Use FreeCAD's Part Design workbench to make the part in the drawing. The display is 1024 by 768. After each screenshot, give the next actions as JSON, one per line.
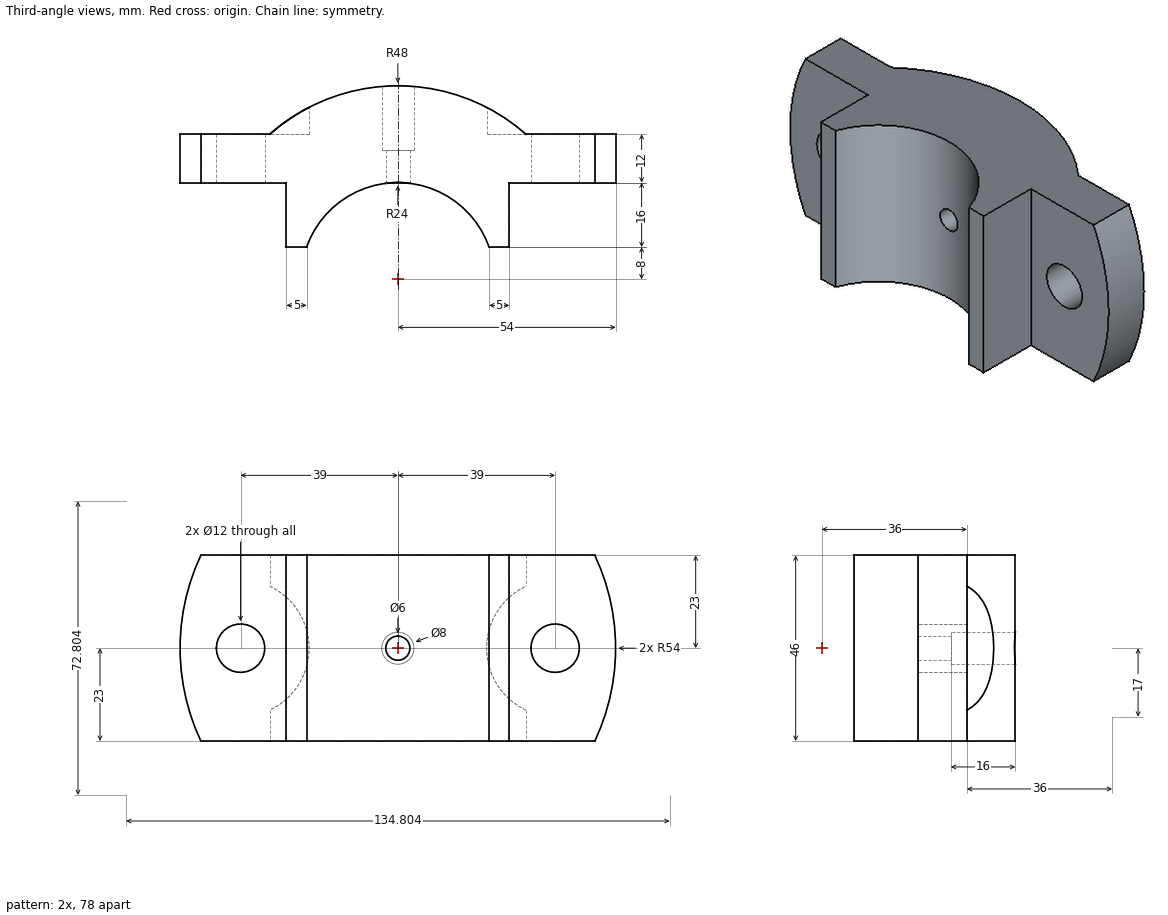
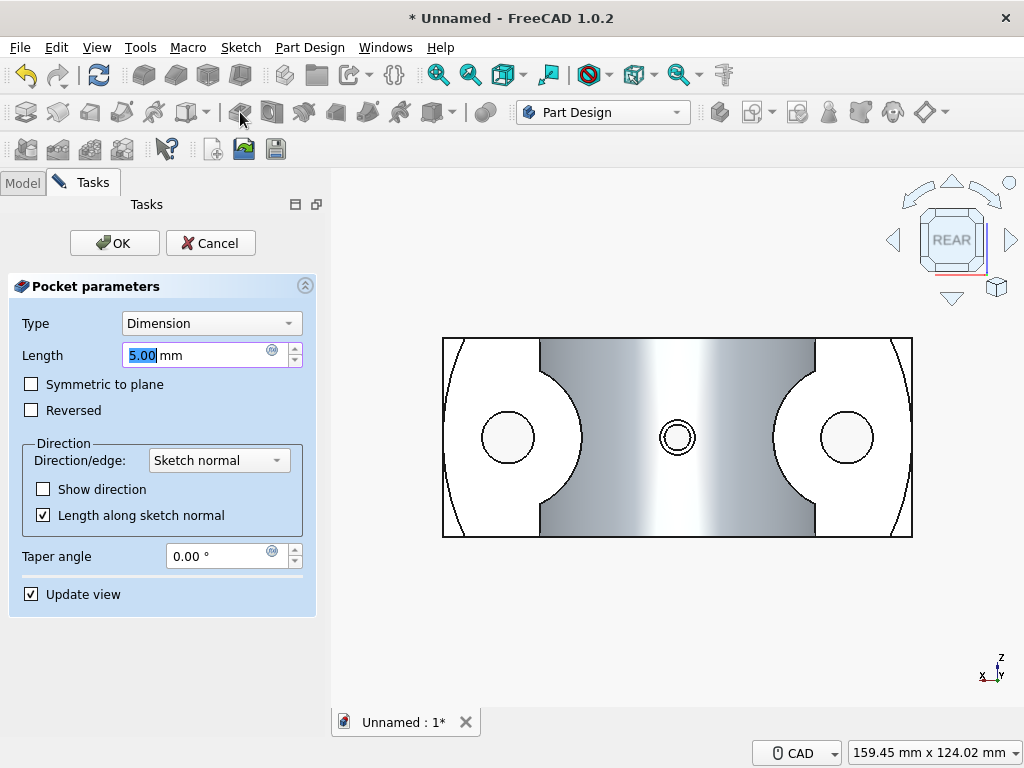
{"action": "left_click", "coordinate": [212, 324]}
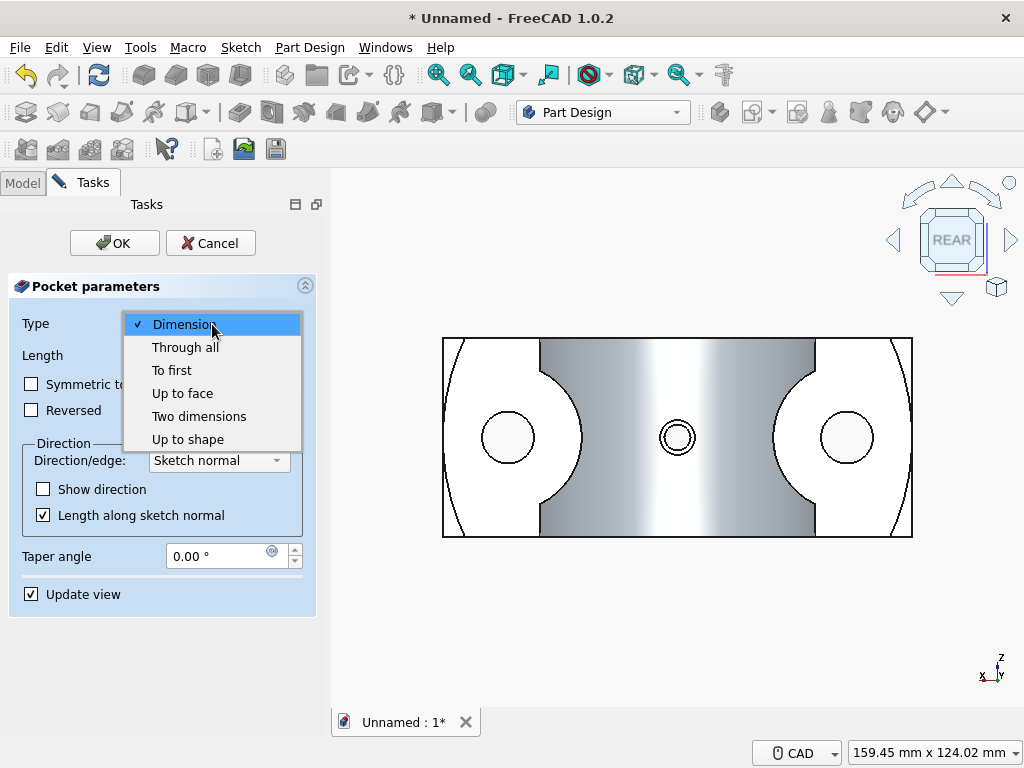
{"action": "left_click", "coordinate": [212, 348]}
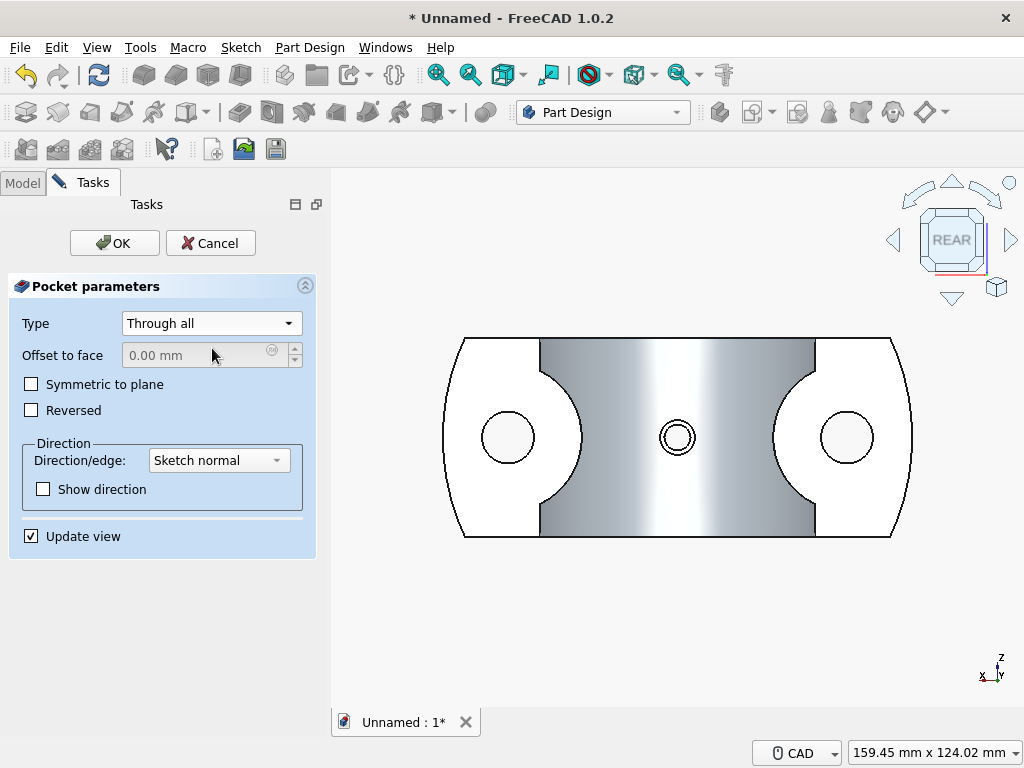
{"action": "left_click", "coordinate": [115, 243]}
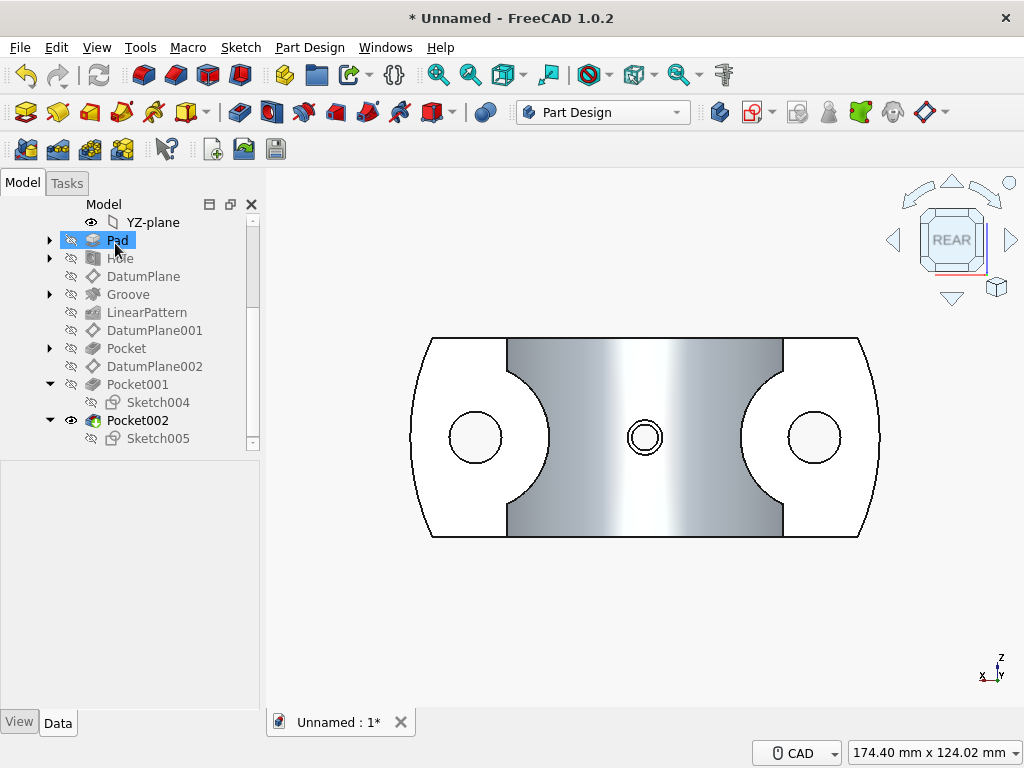
{"action": "key", "text": "0"}